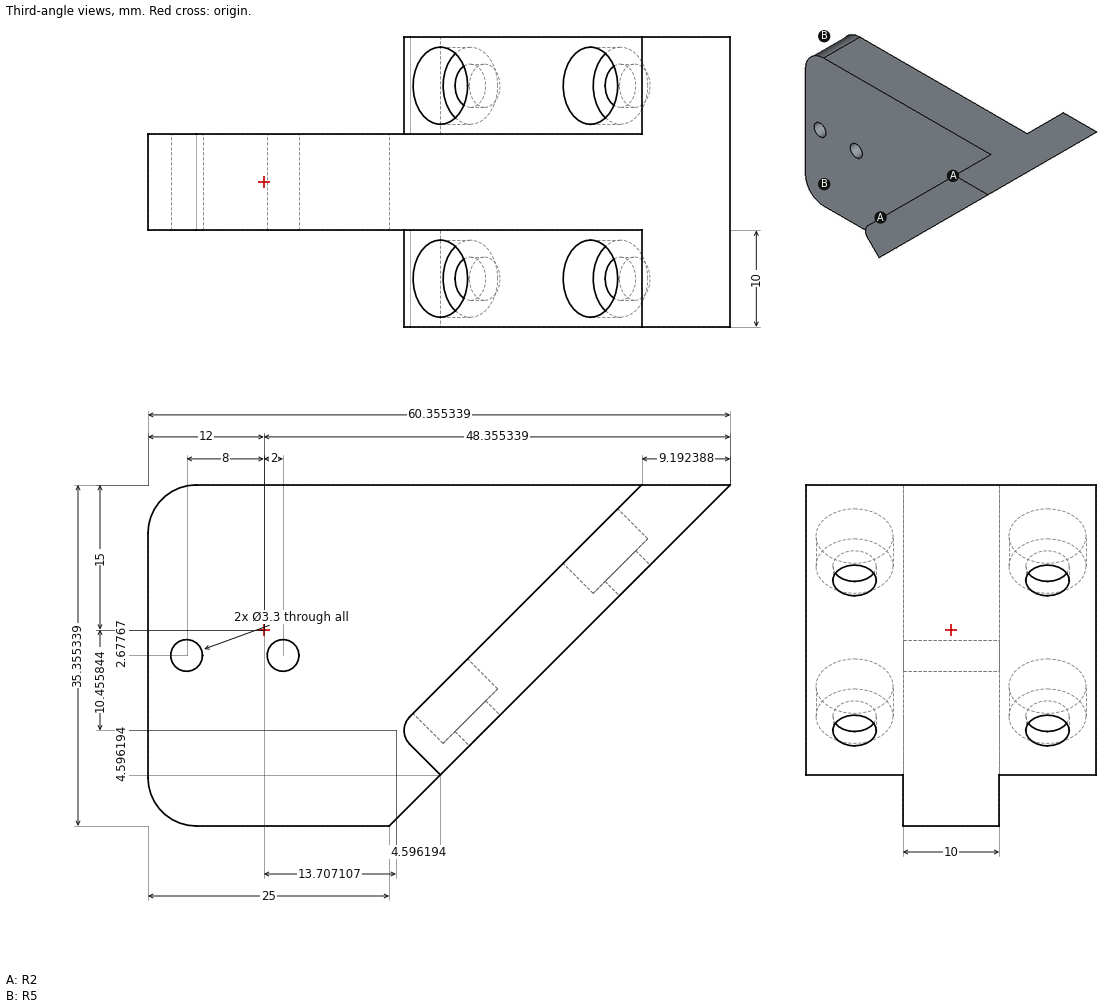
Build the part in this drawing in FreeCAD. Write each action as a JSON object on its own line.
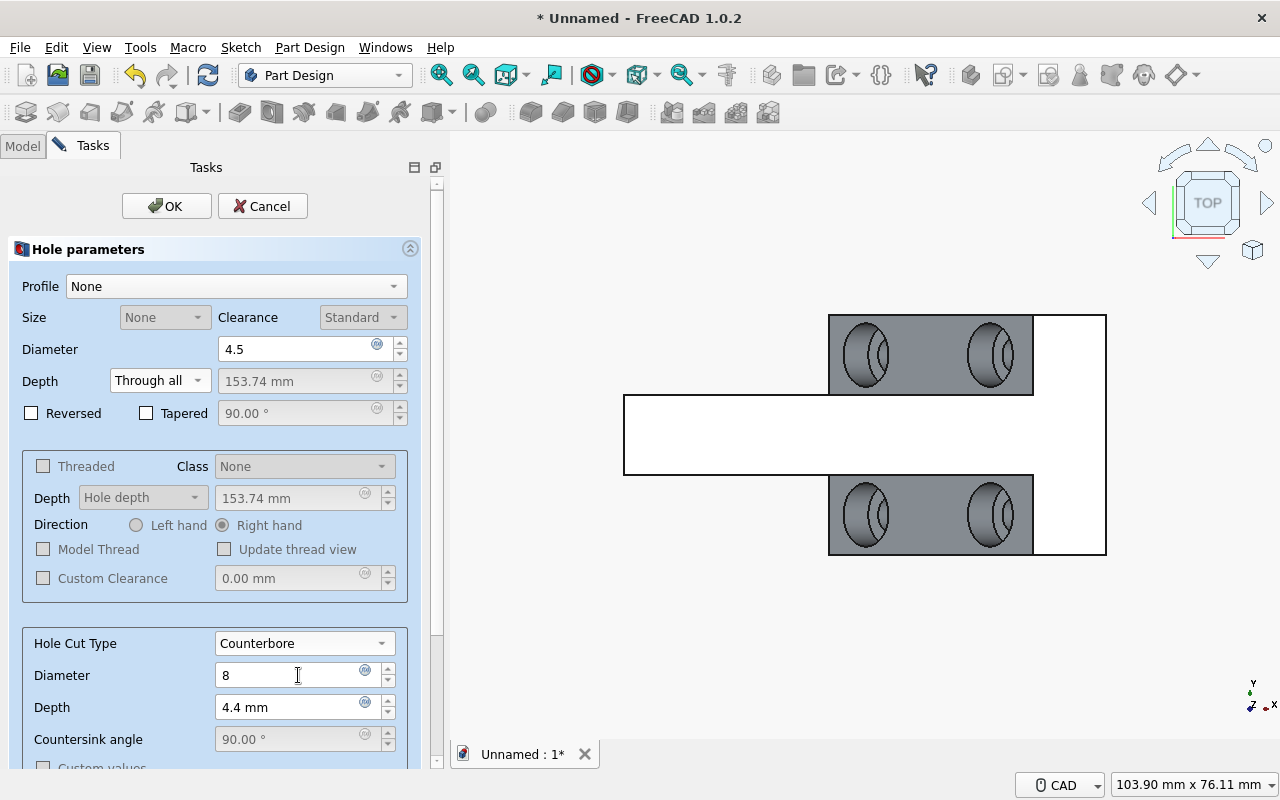
{"action": "left_click", "coordinate": [167, 206]}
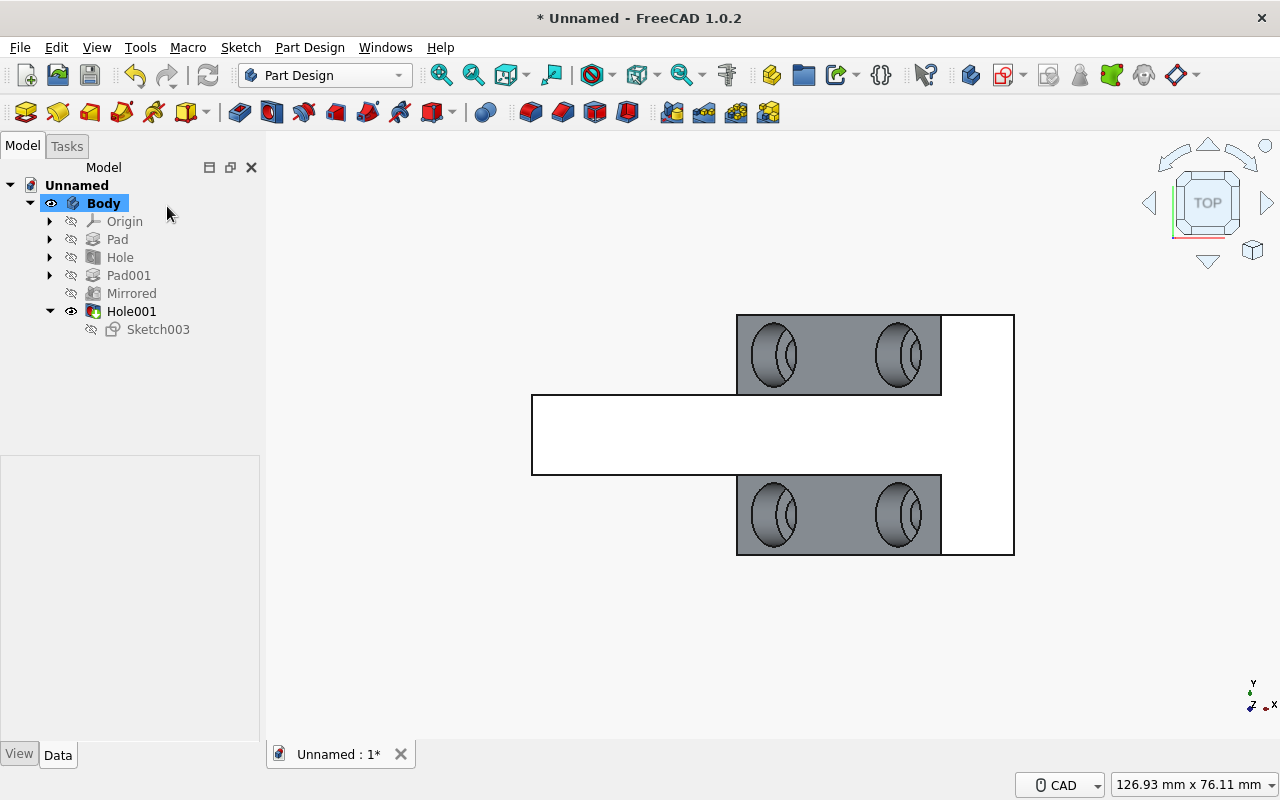
{"action": "key", "text": "0"}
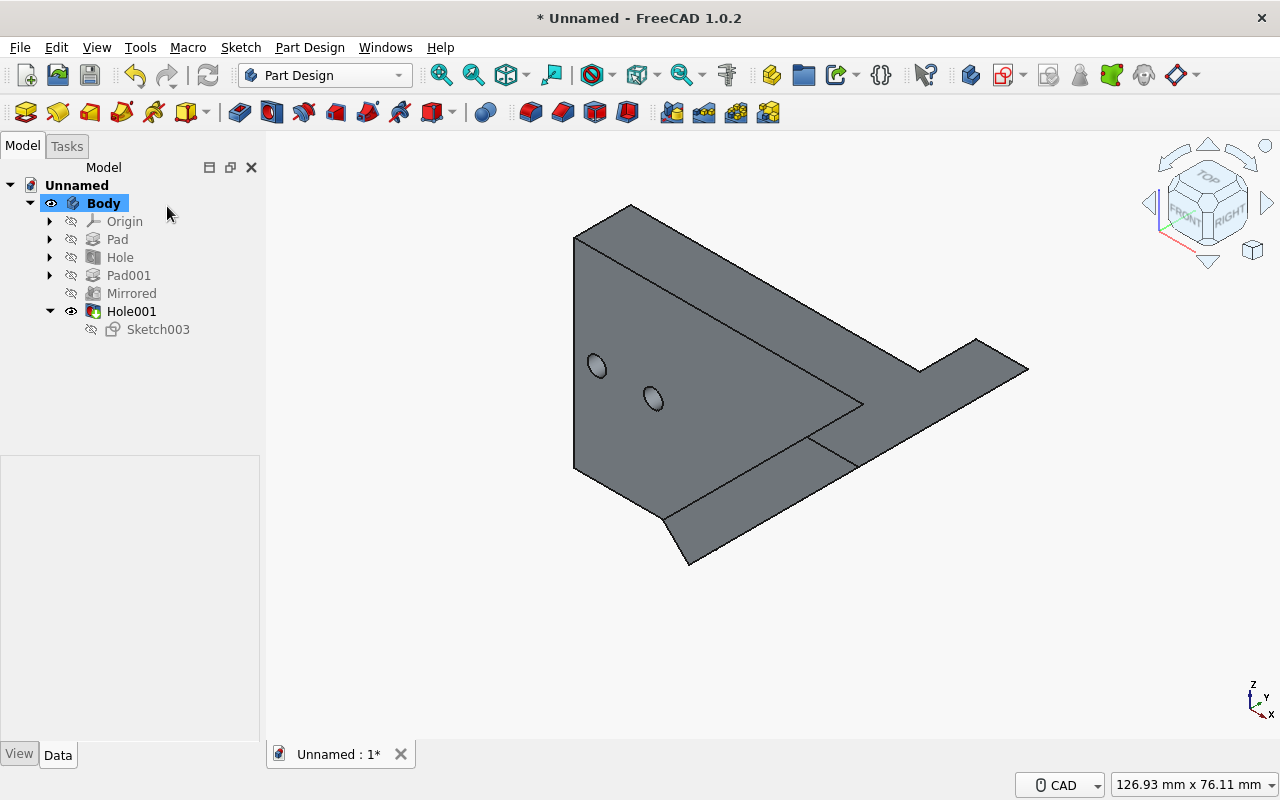
{"action": "key", "text": "2"}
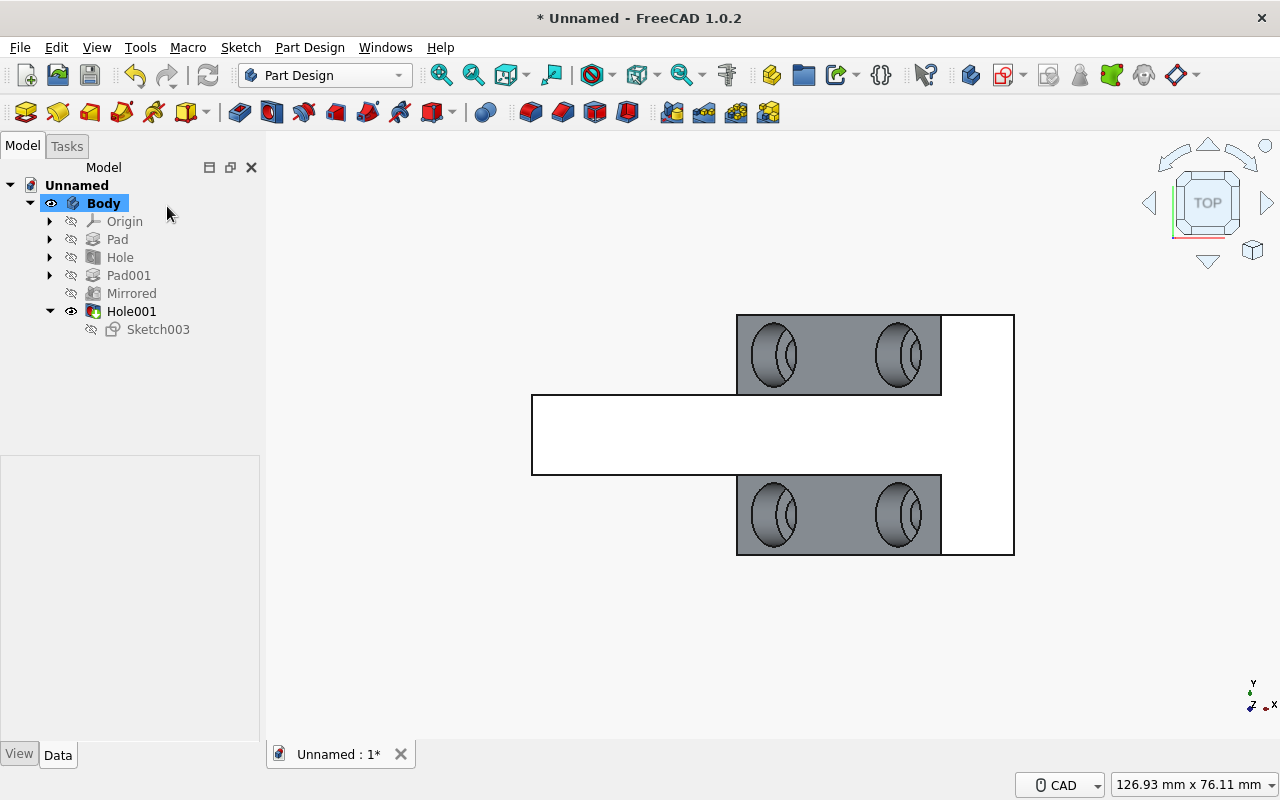
{"action": "key", "text": "1"}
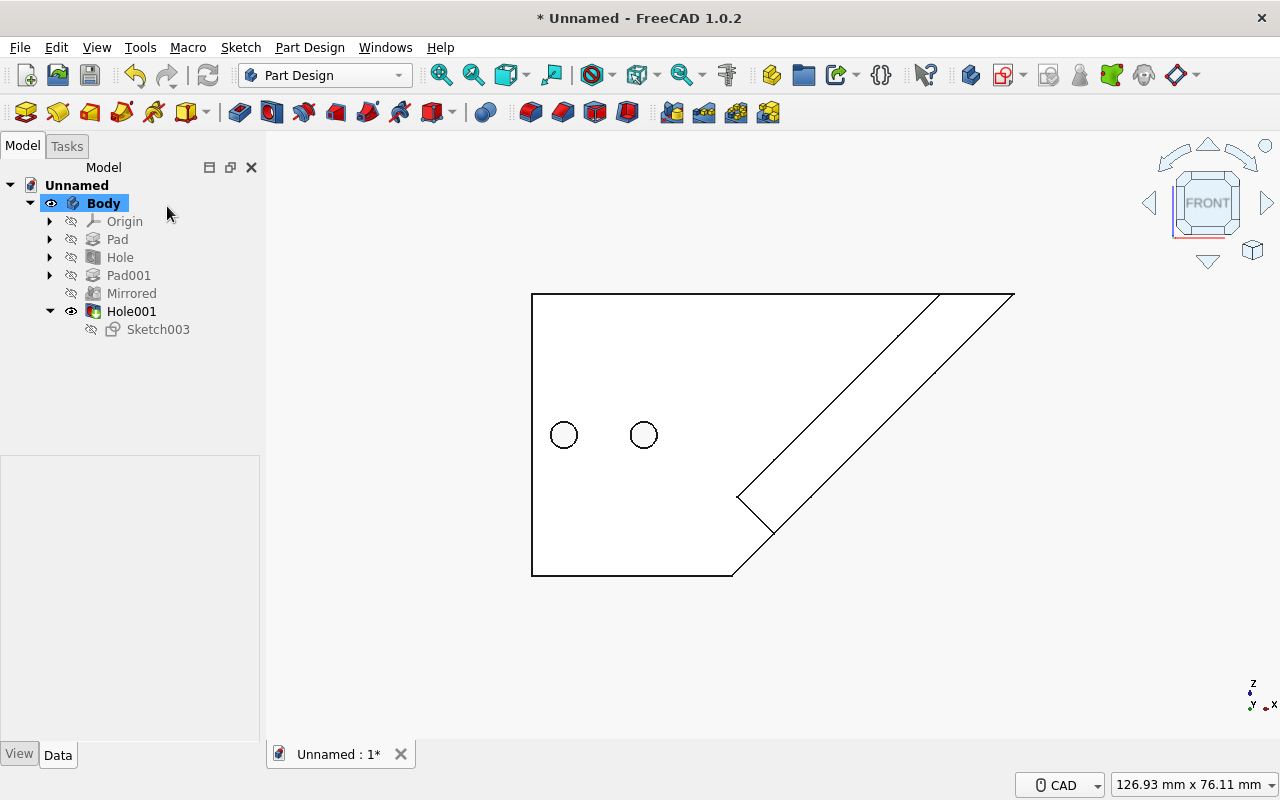
{"action": "key", "text": "3"}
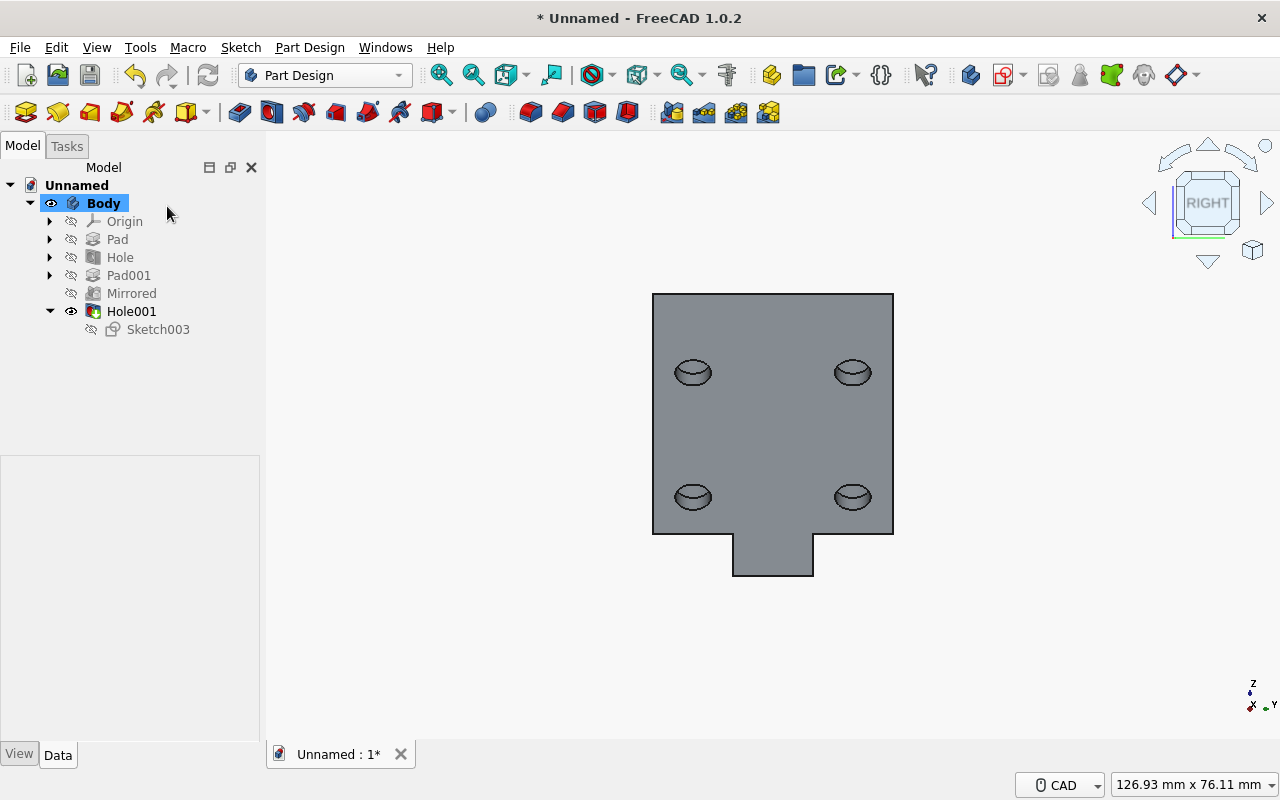
{"action": "key", "text": "5"}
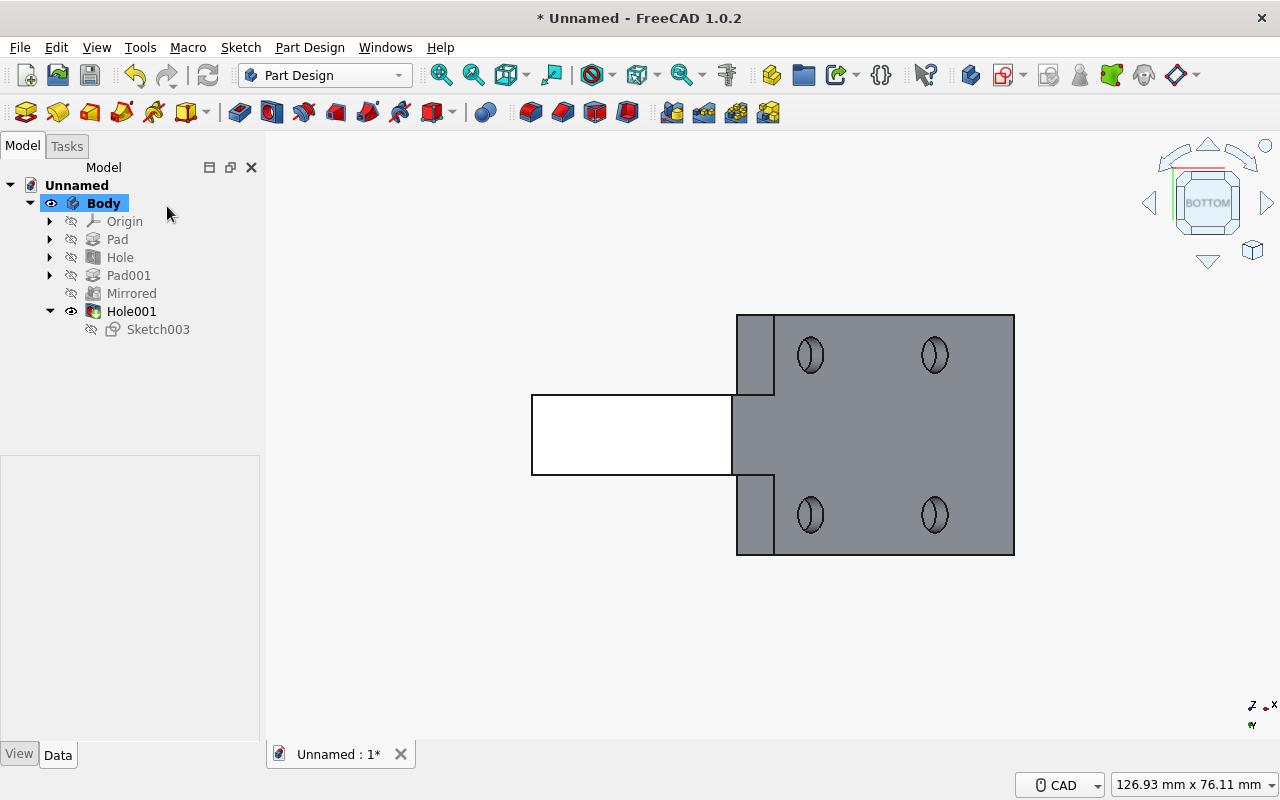
{"action": "key", "text": "4"}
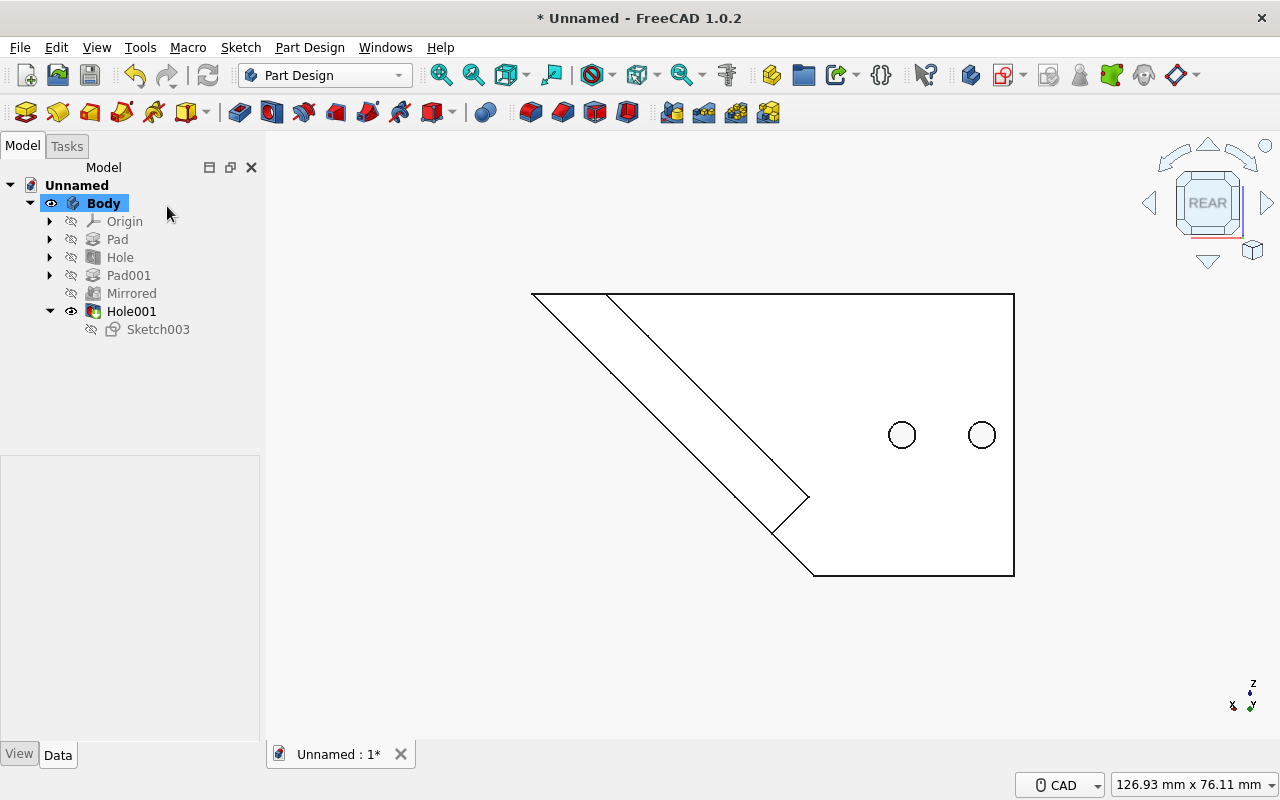
{"action": "key", "text": "6"}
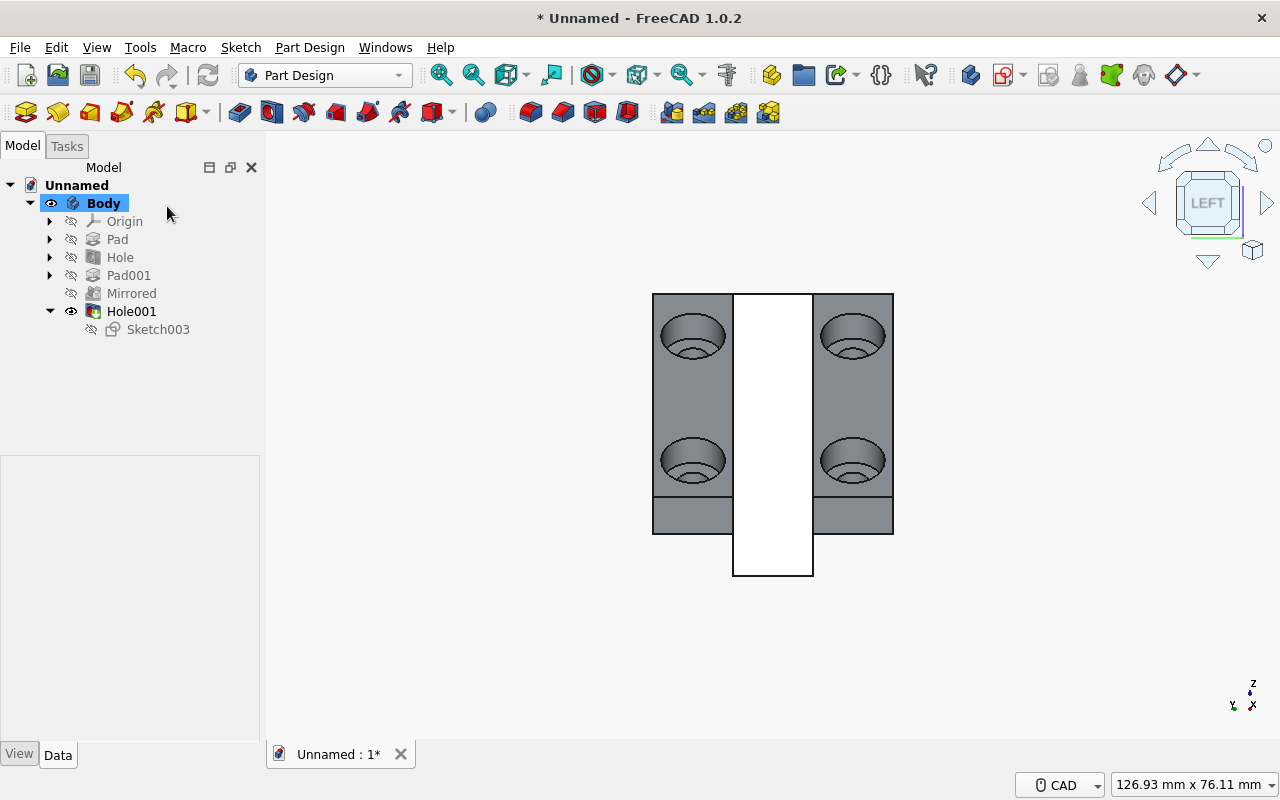
{"action": "left_click", "coordinate": [853, 496]}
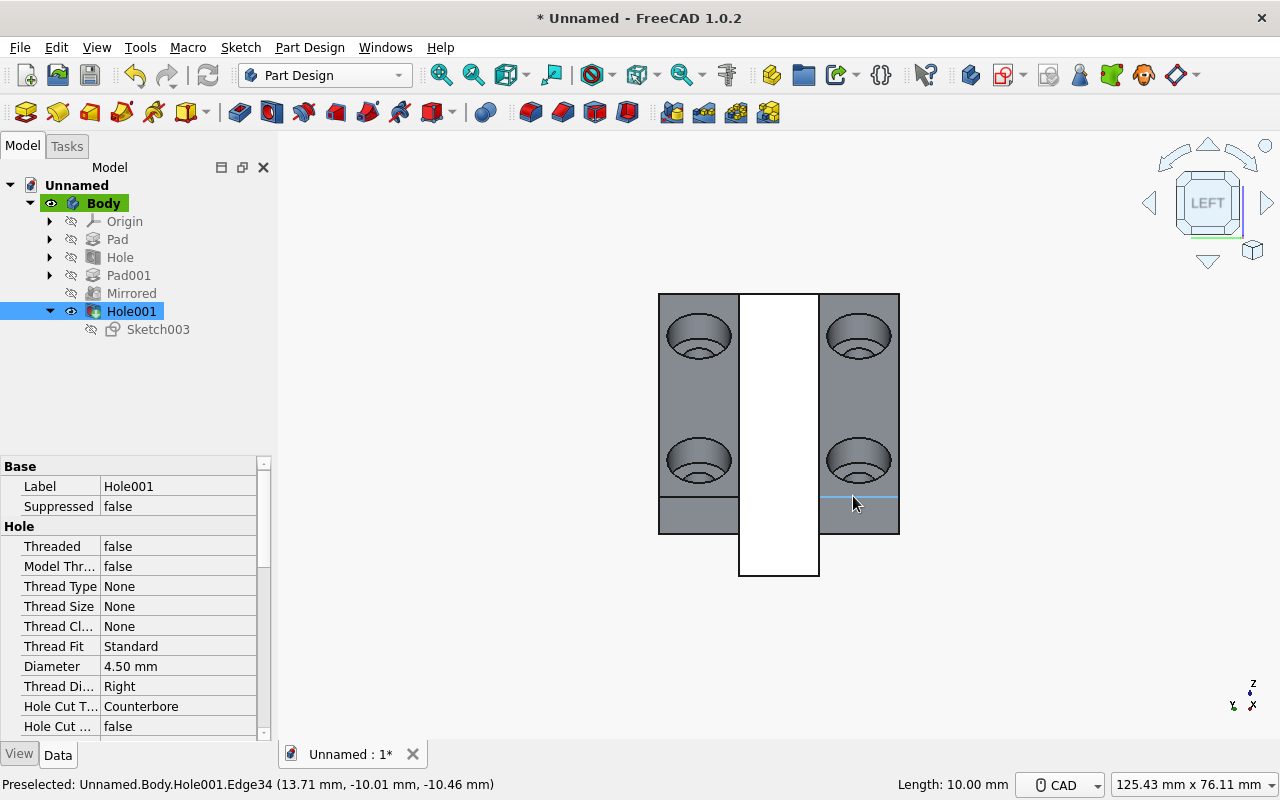
{"action": "left_click", "coordinate": [699, 496], "text": "ctrl"}